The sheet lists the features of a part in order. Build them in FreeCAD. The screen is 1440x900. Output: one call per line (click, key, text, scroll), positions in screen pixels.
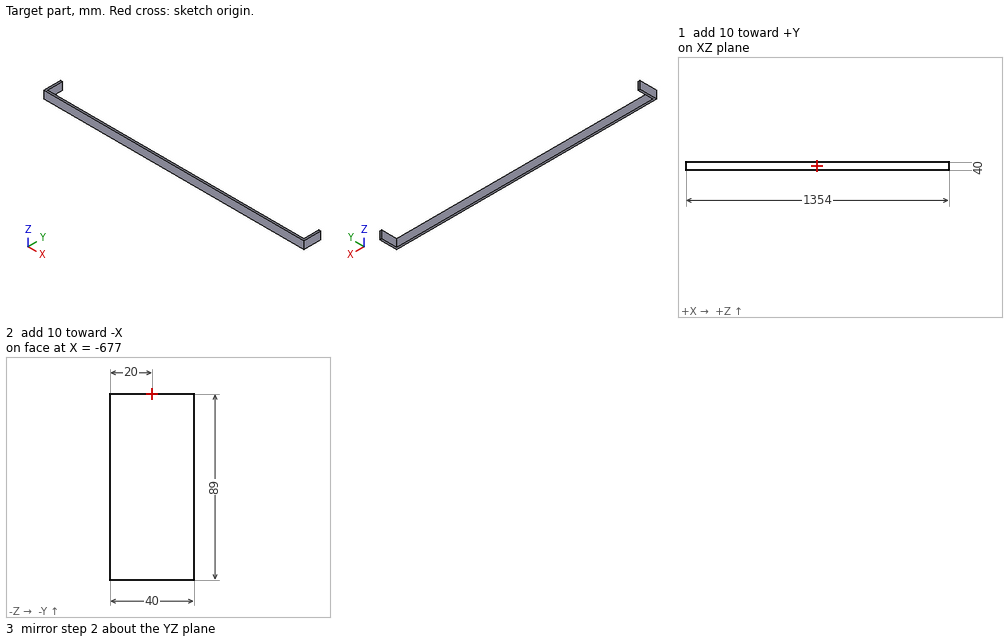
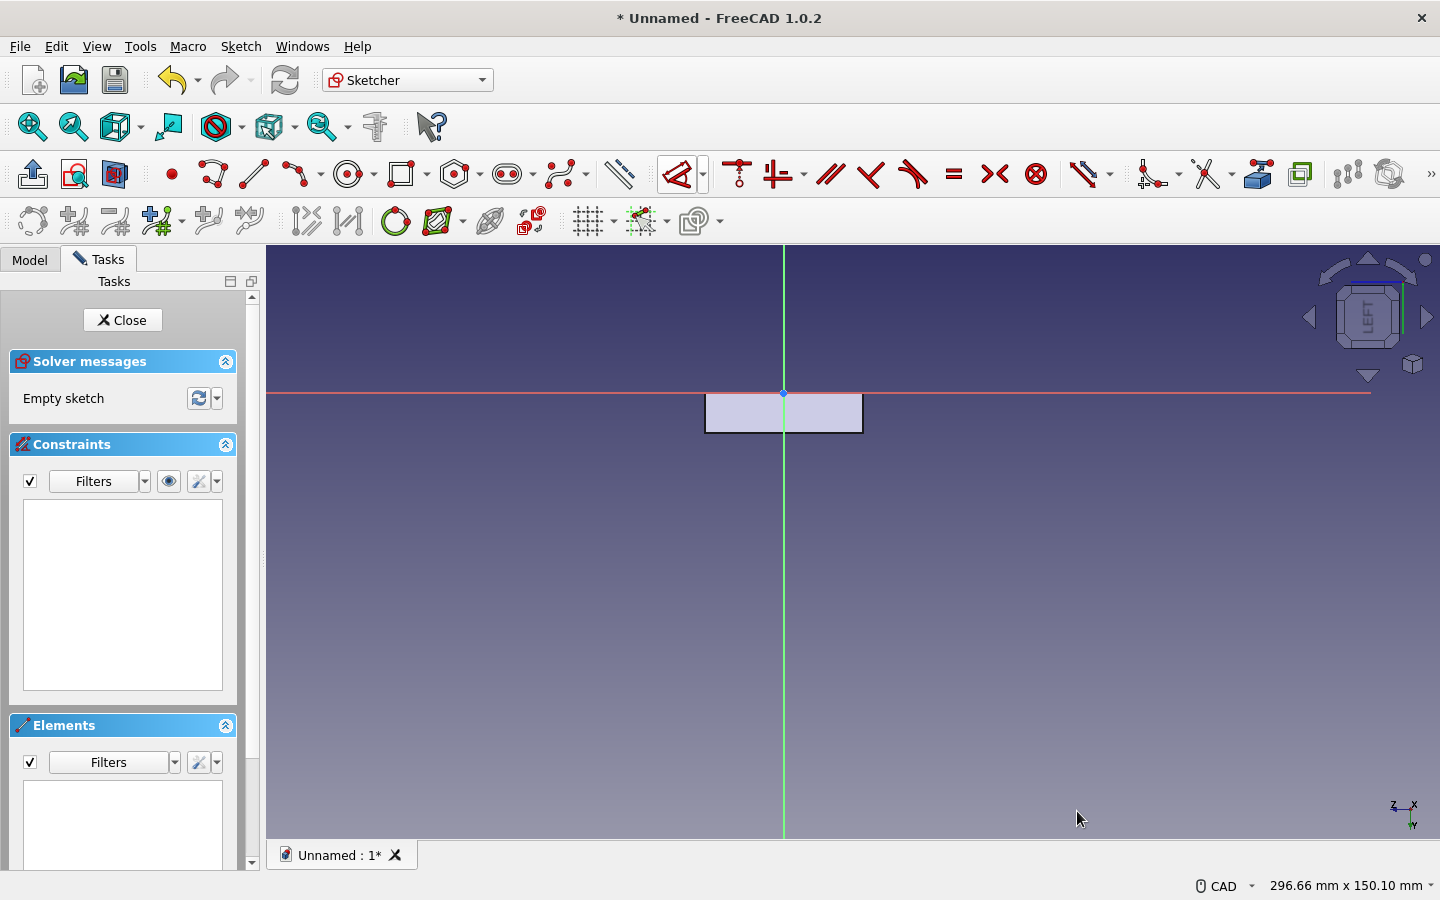
key(g)
key(r)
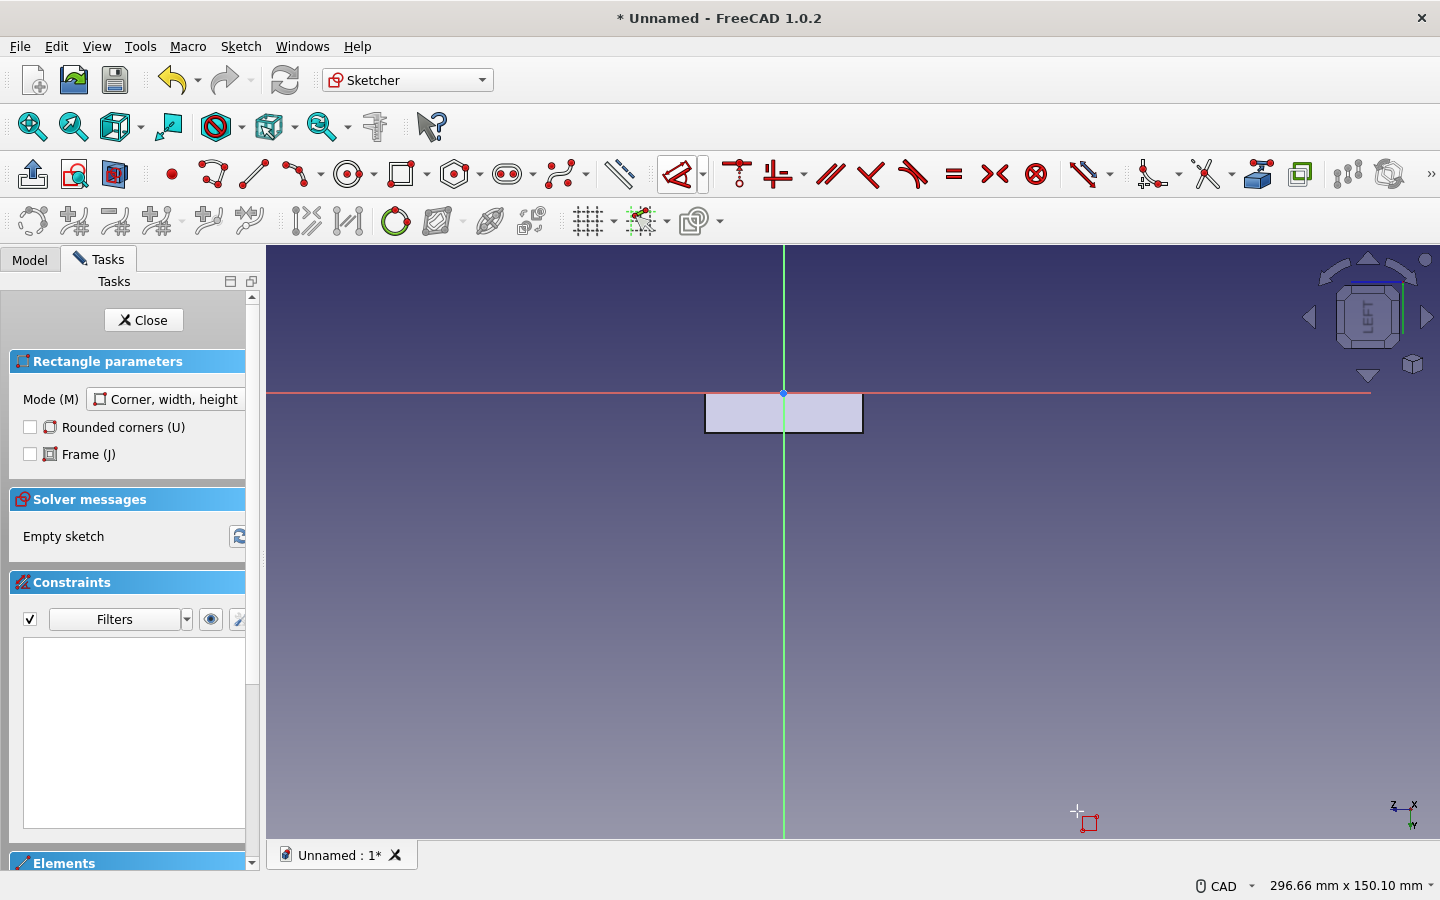
click(705, 393)
move(863, 745)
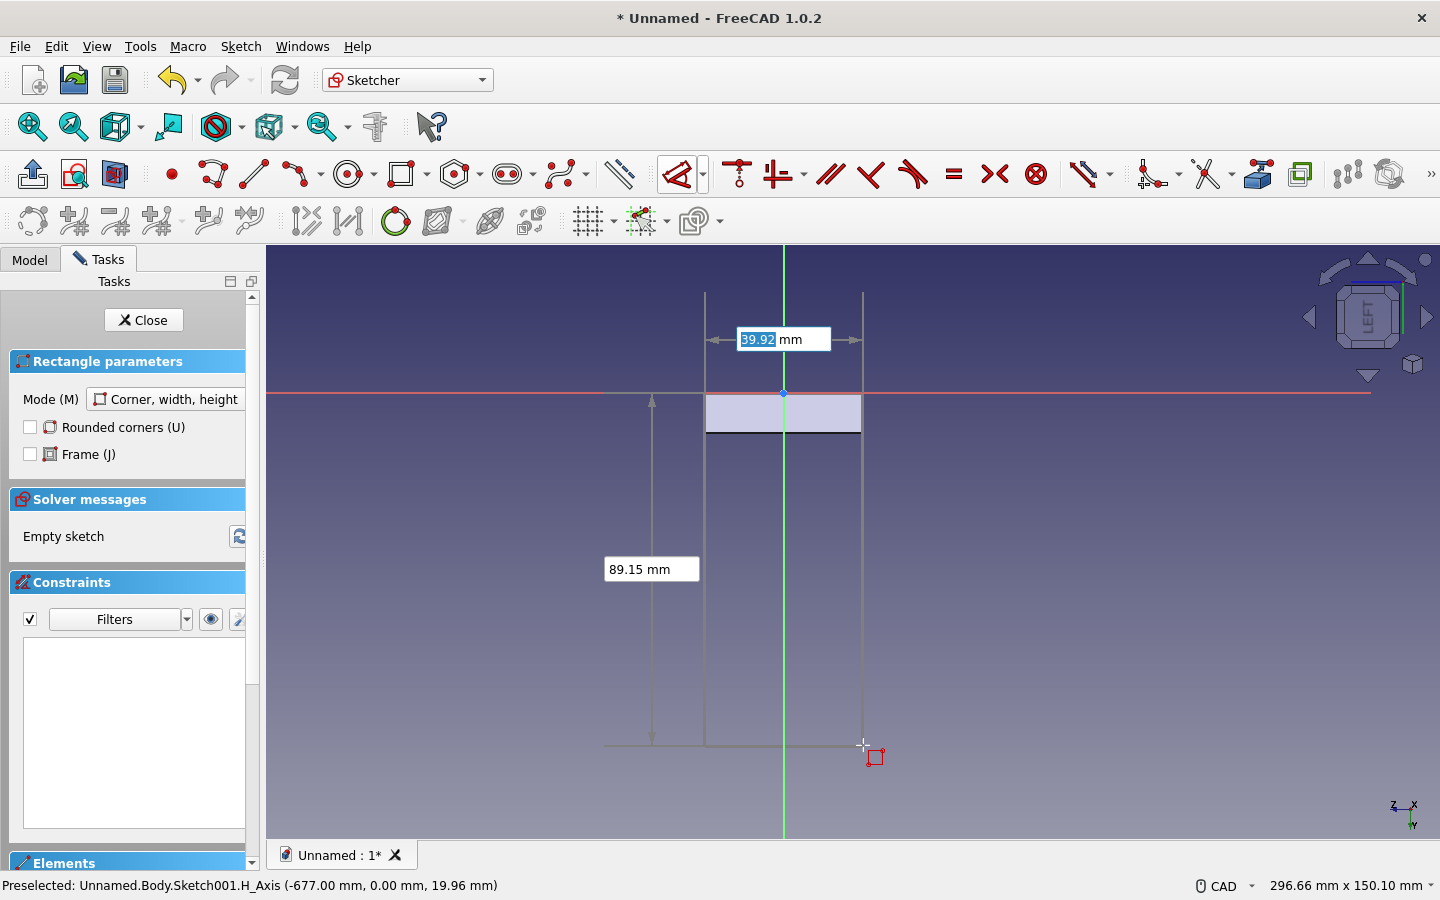
text(40)
key(Tab)
text(89)
key(Return)
key(Escape)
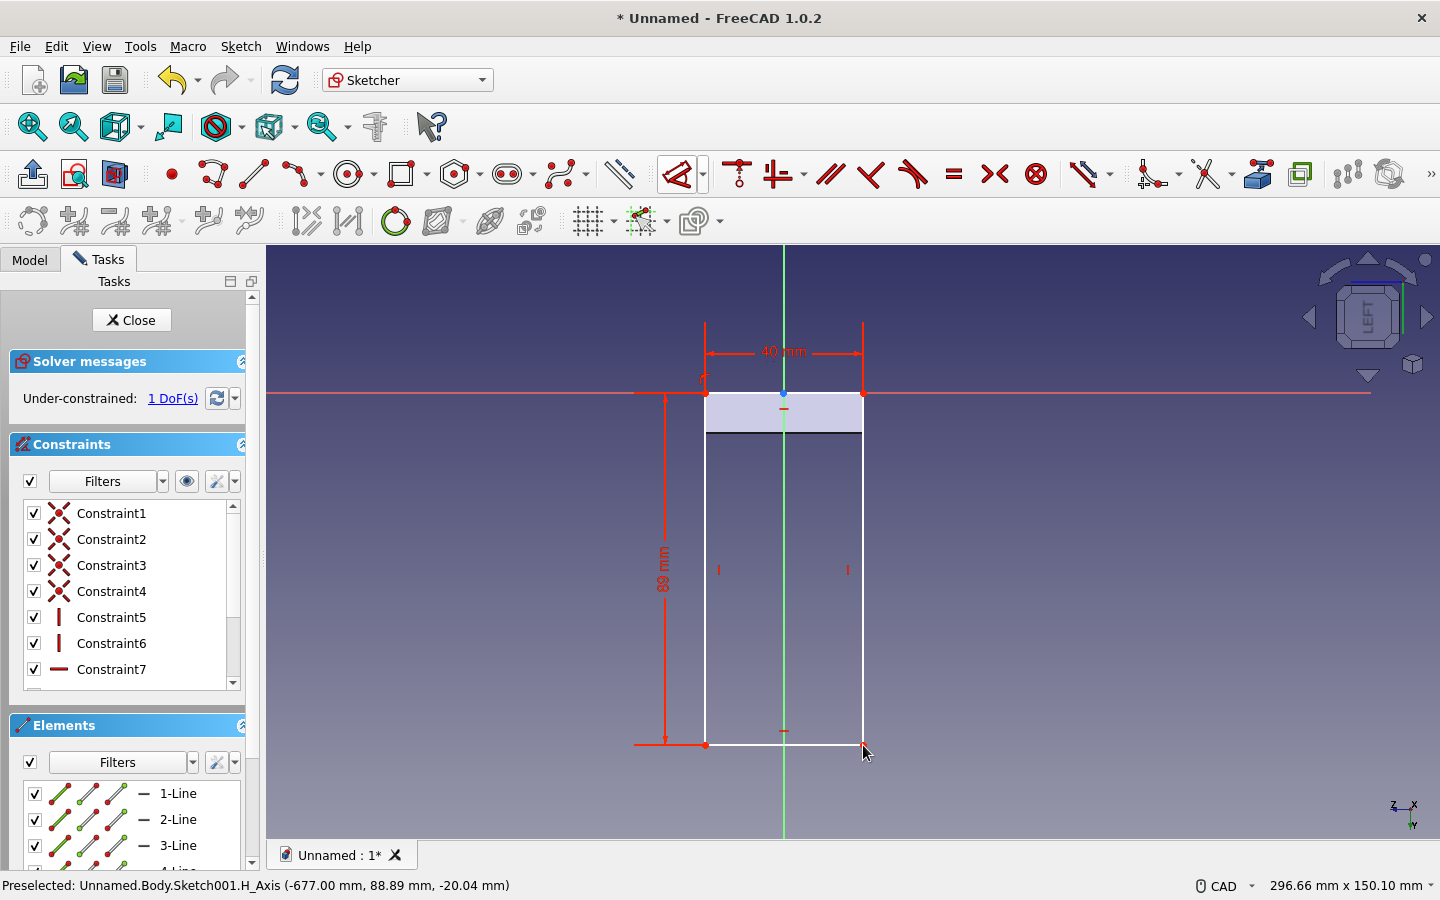
click(705, 393)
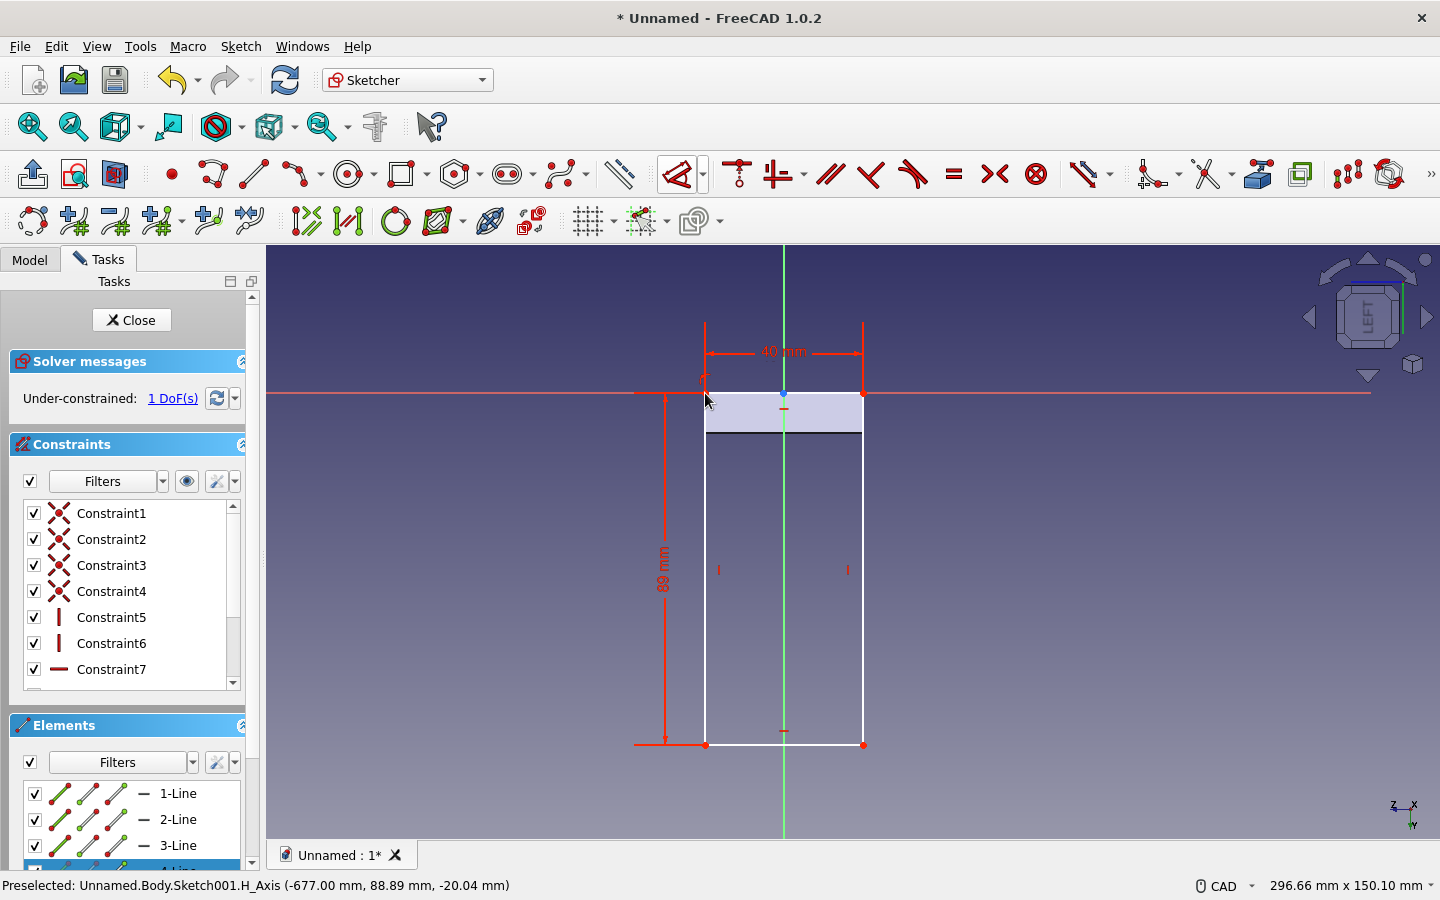
key(l)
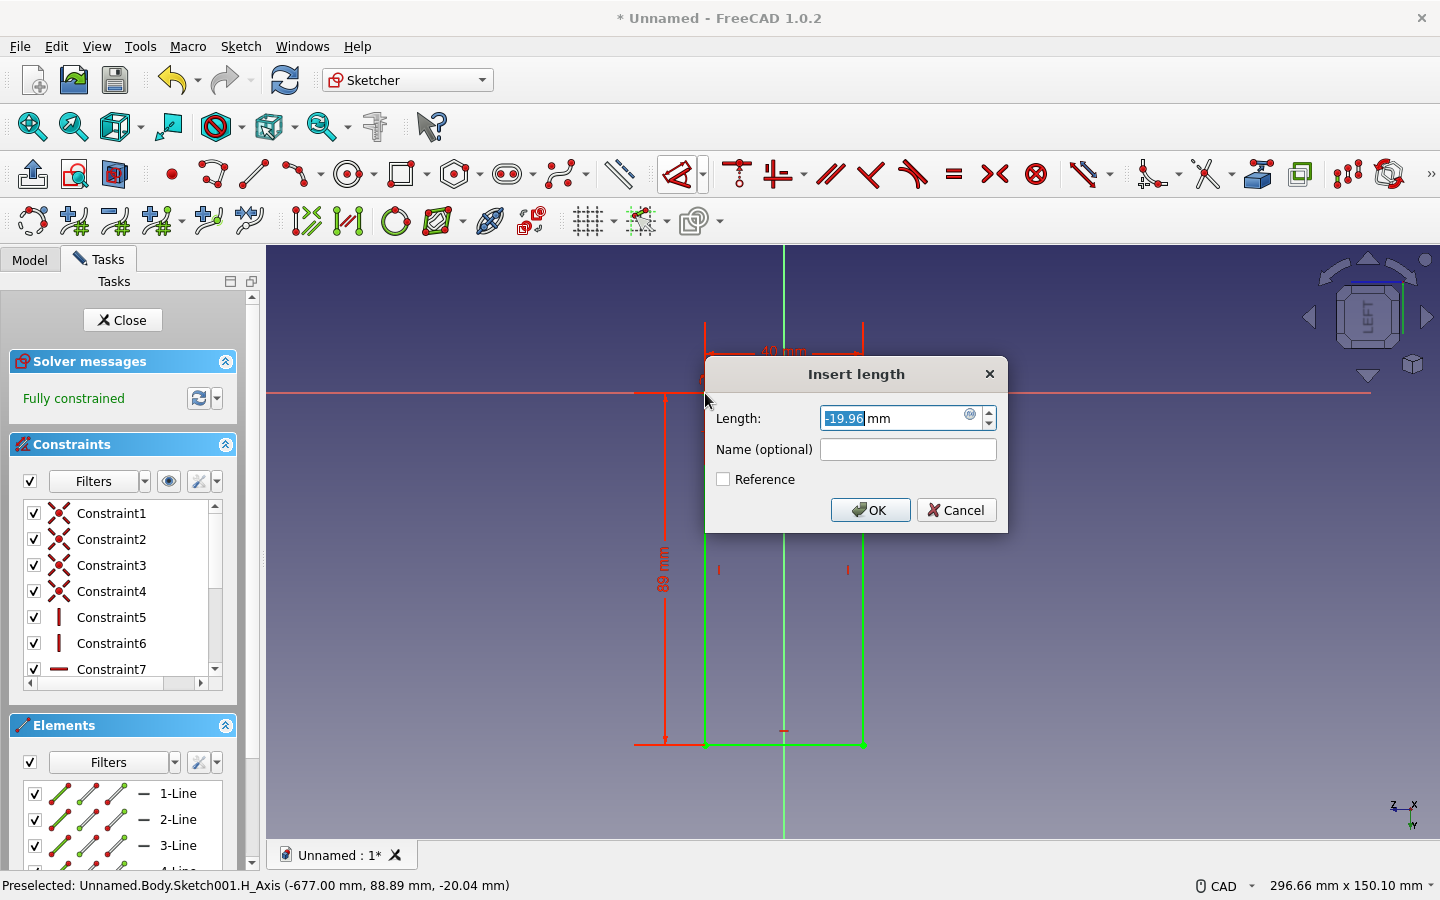
text(-20)
key(Return)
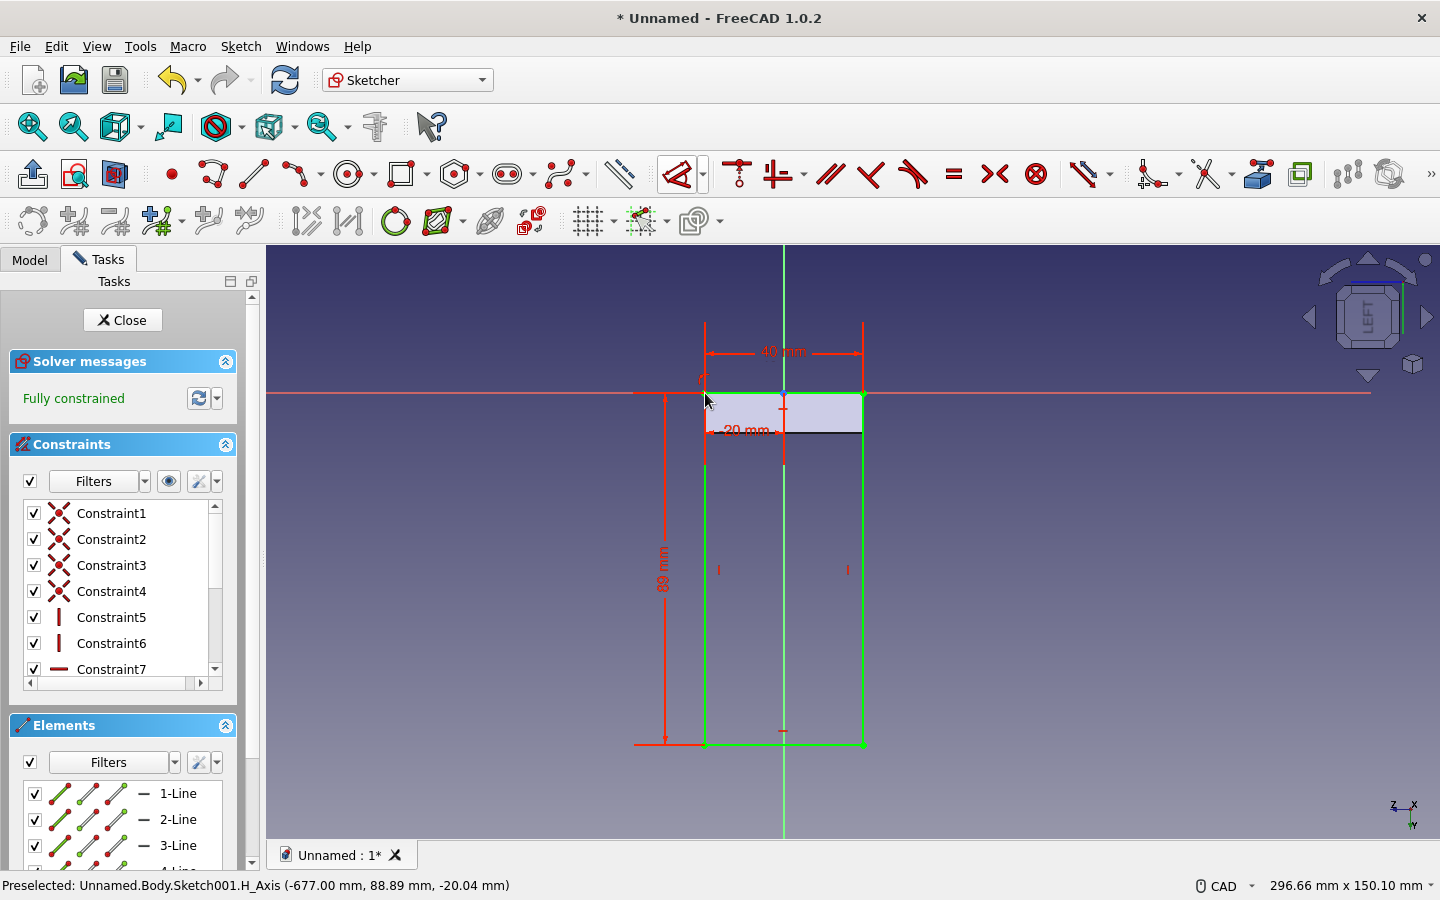
click(123, 320)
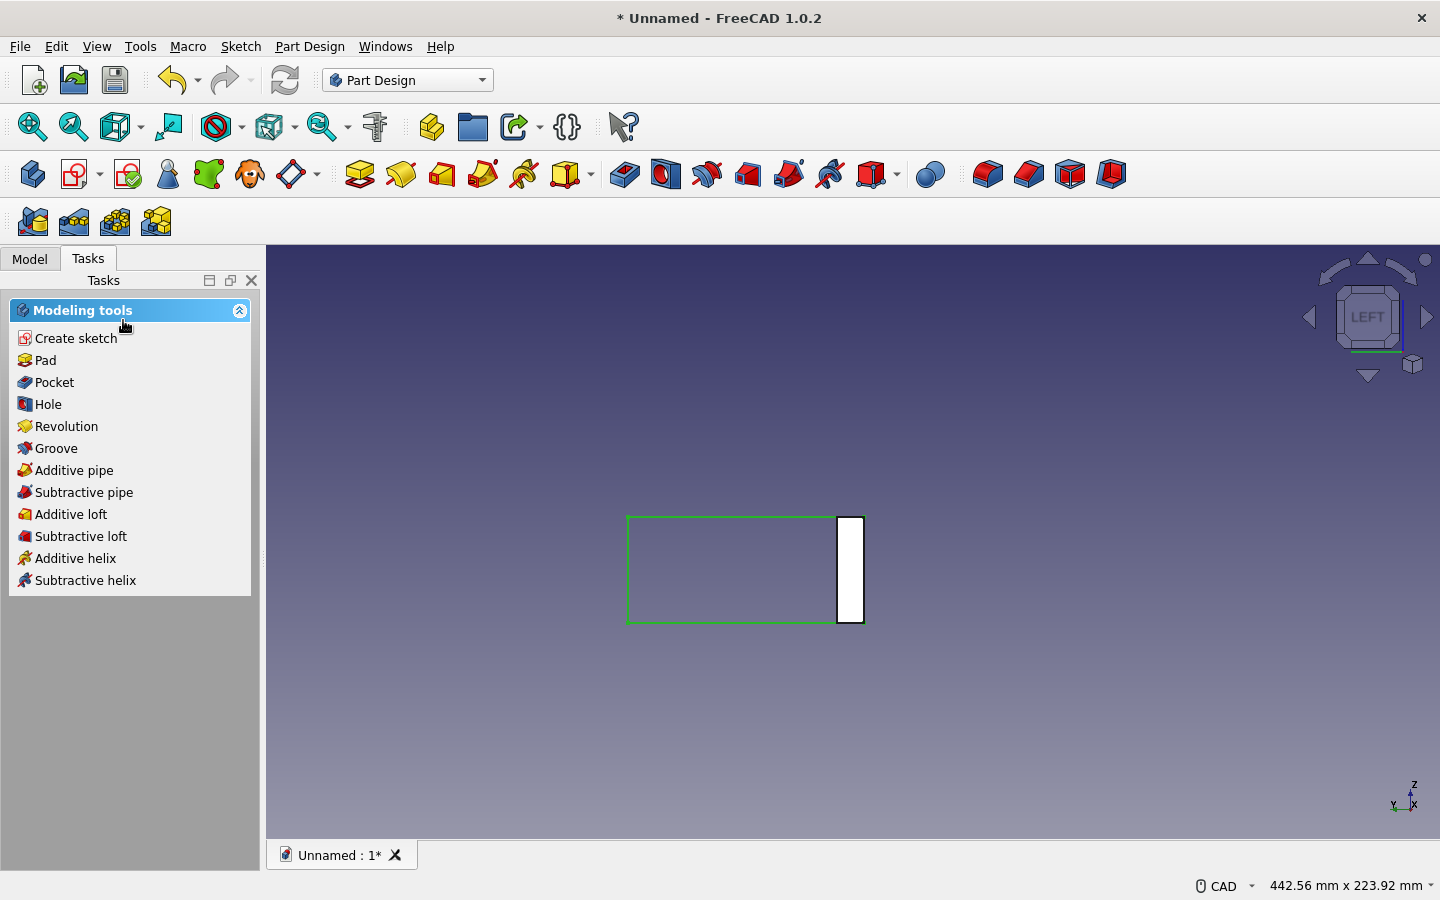
click(360, 174)